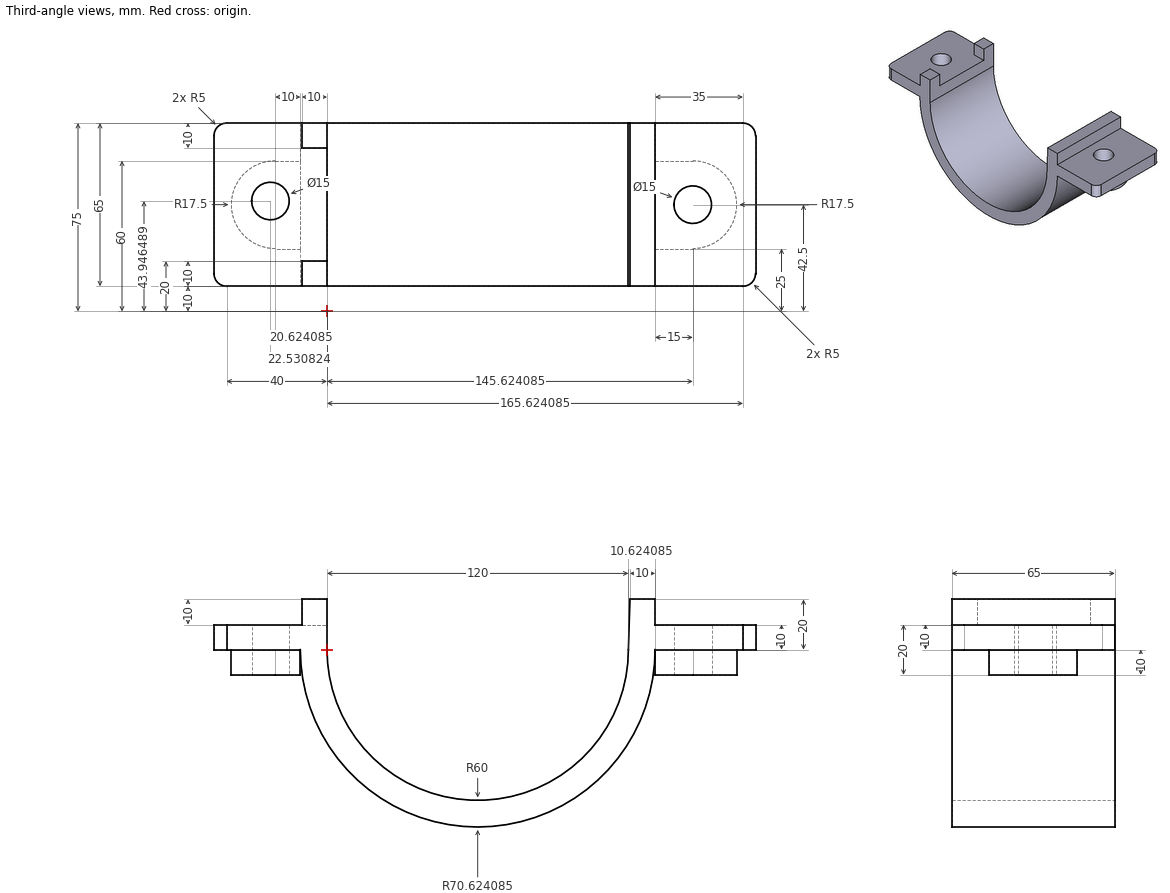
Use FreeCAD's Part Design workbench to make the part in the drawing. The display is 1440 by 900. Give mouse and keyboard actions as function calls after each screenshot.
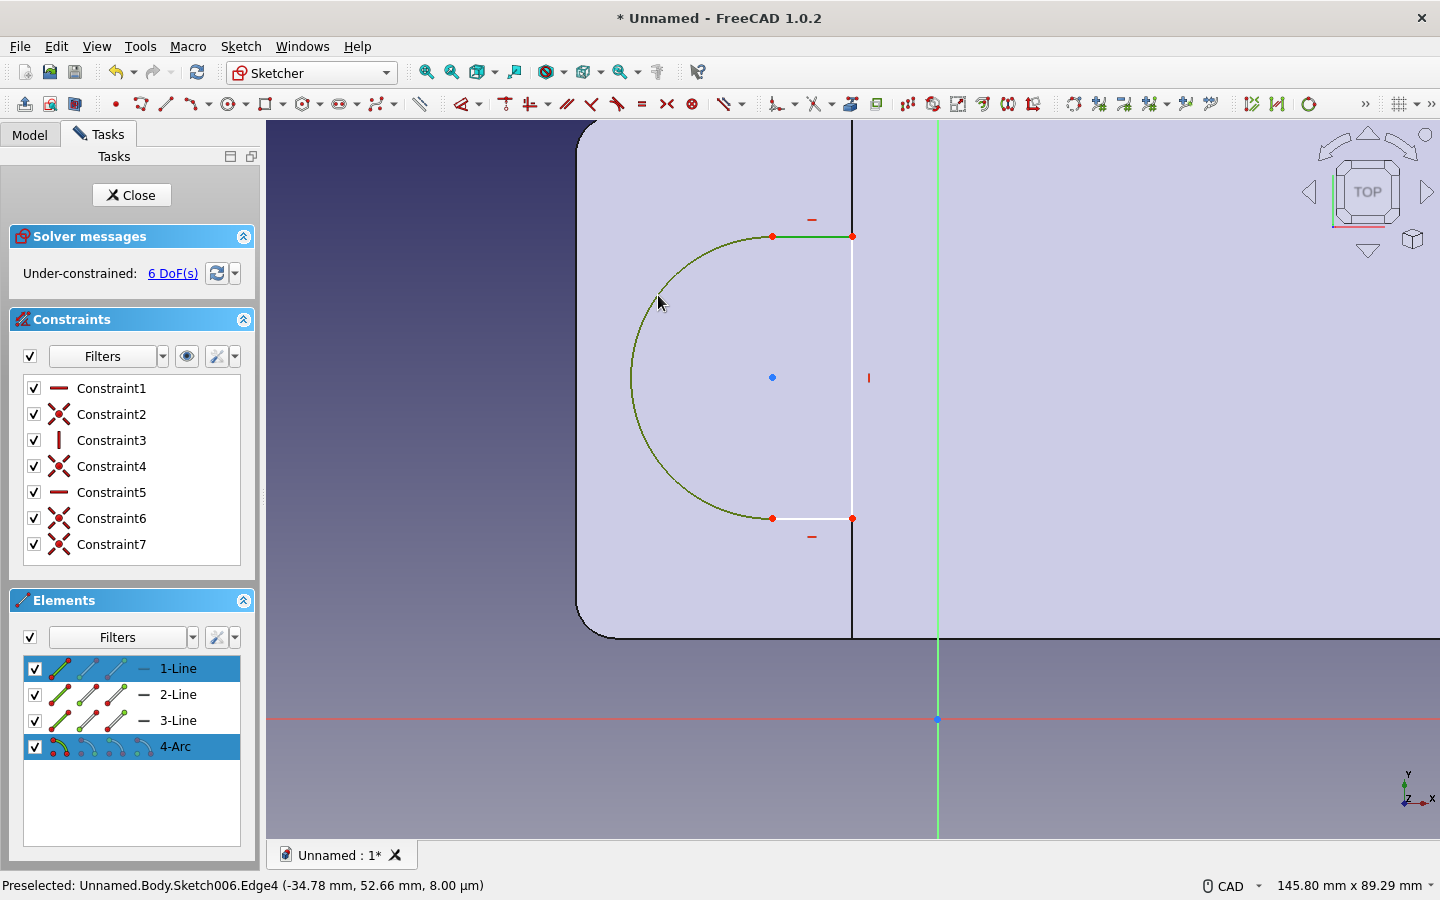
key(t)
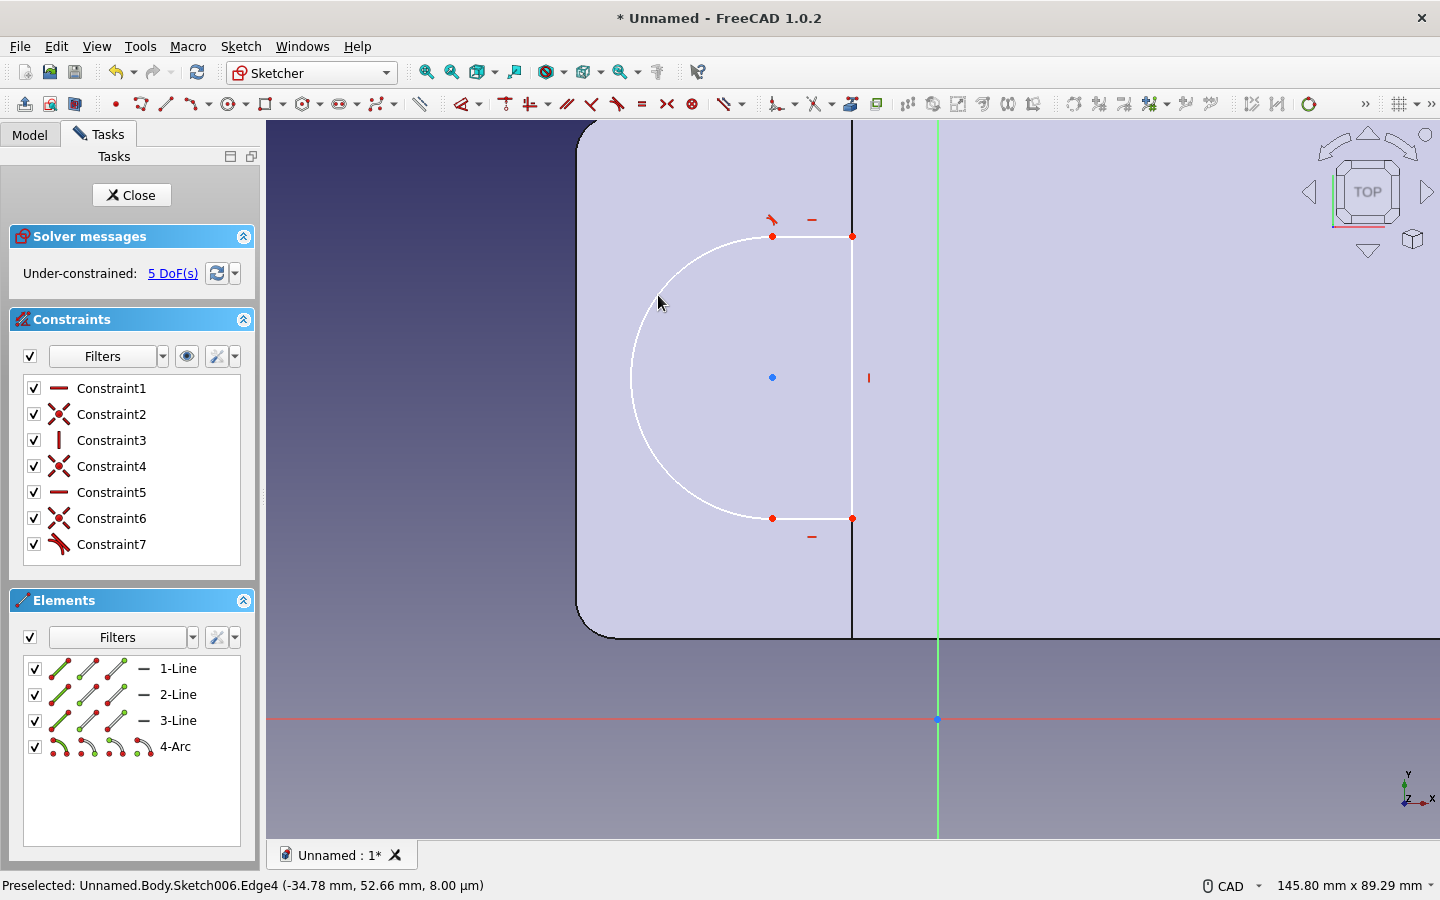
click(828, 519)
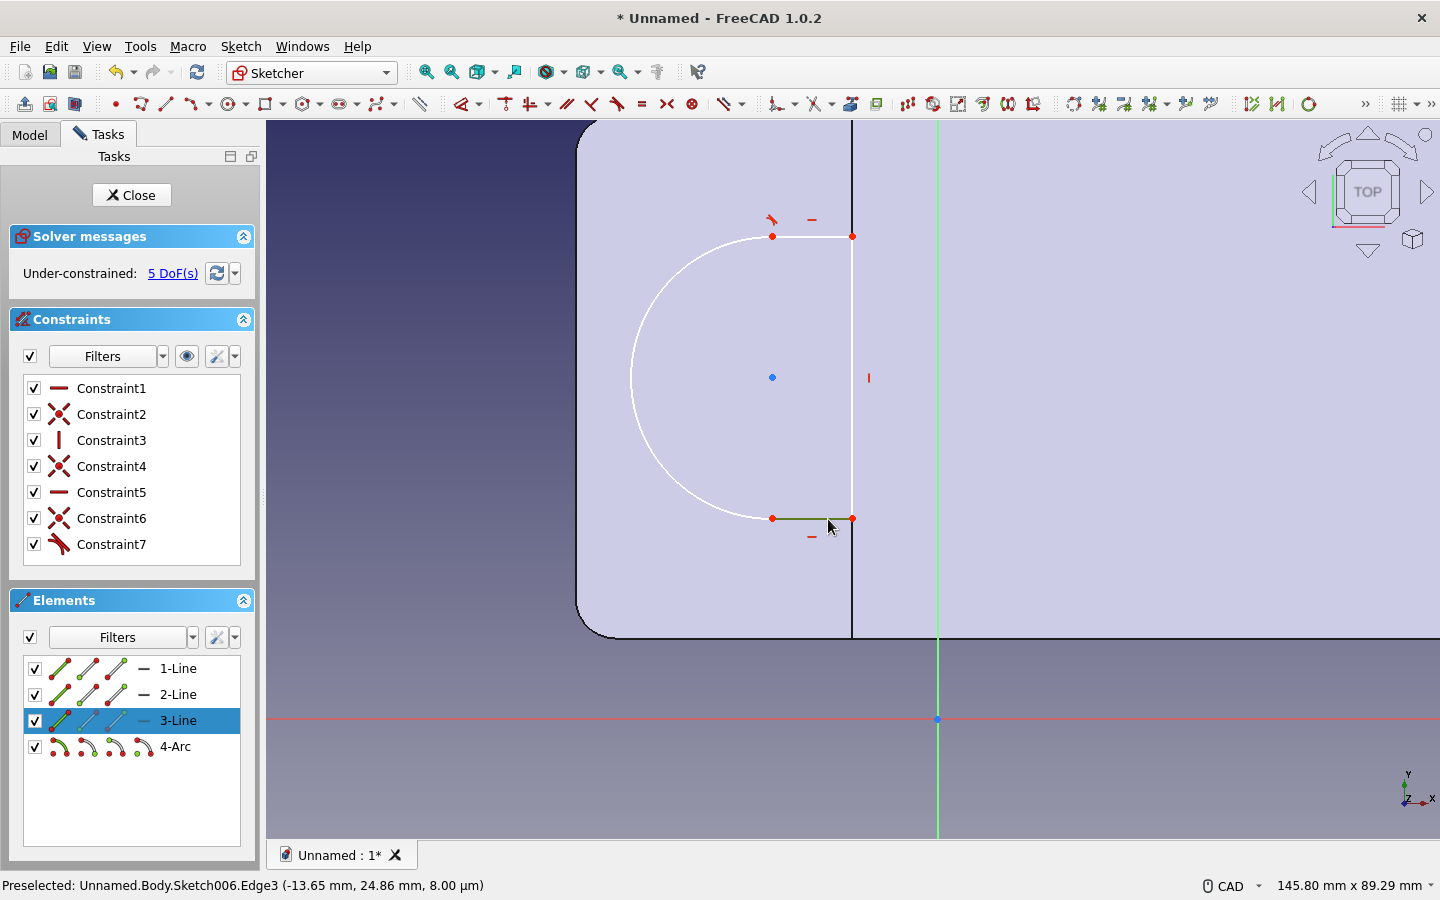
click(658, 295)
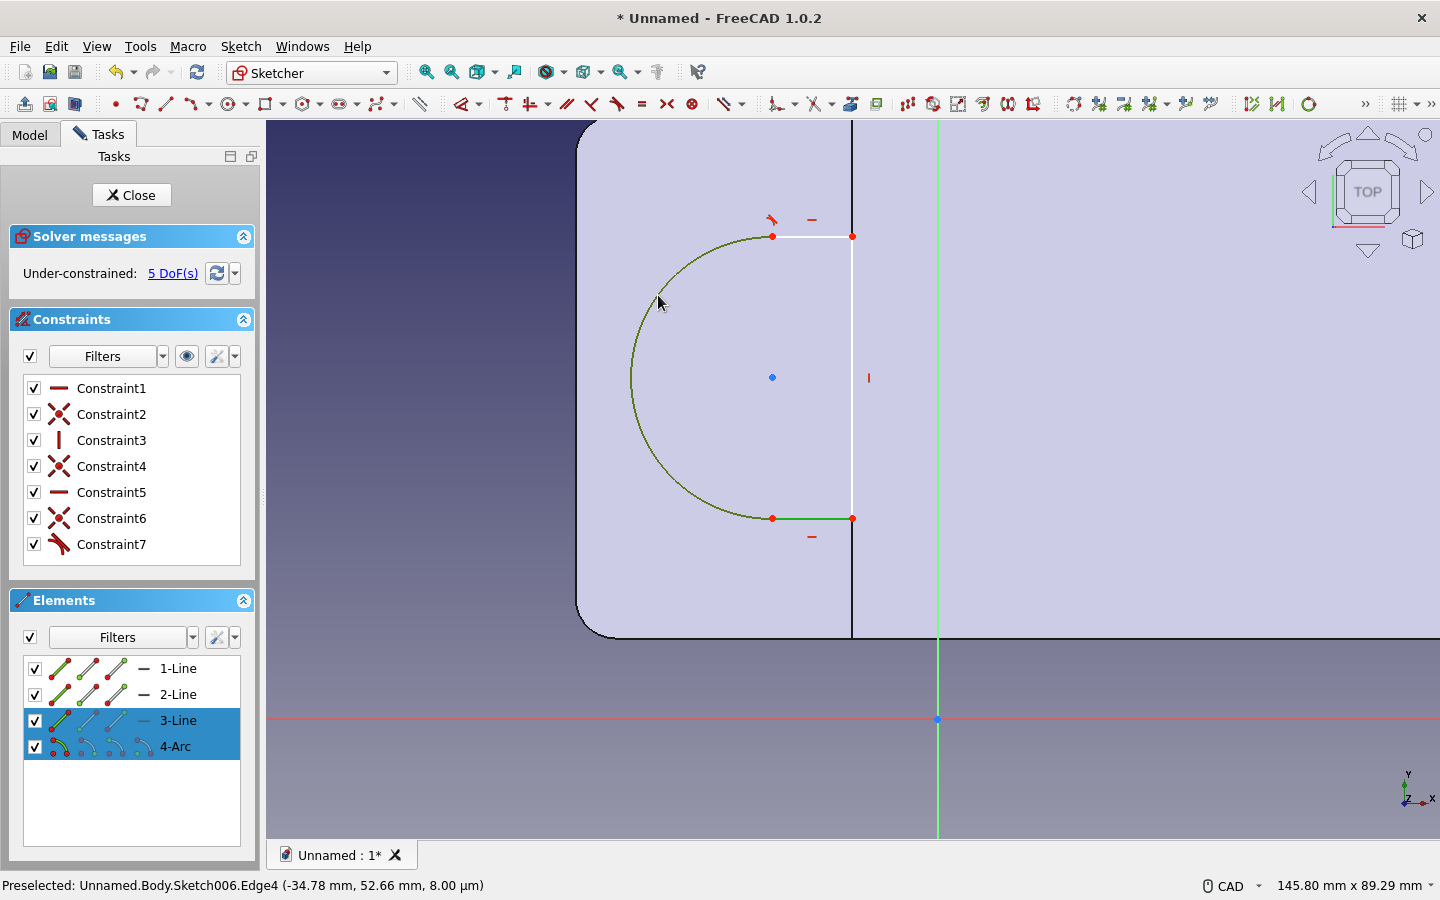
key(t)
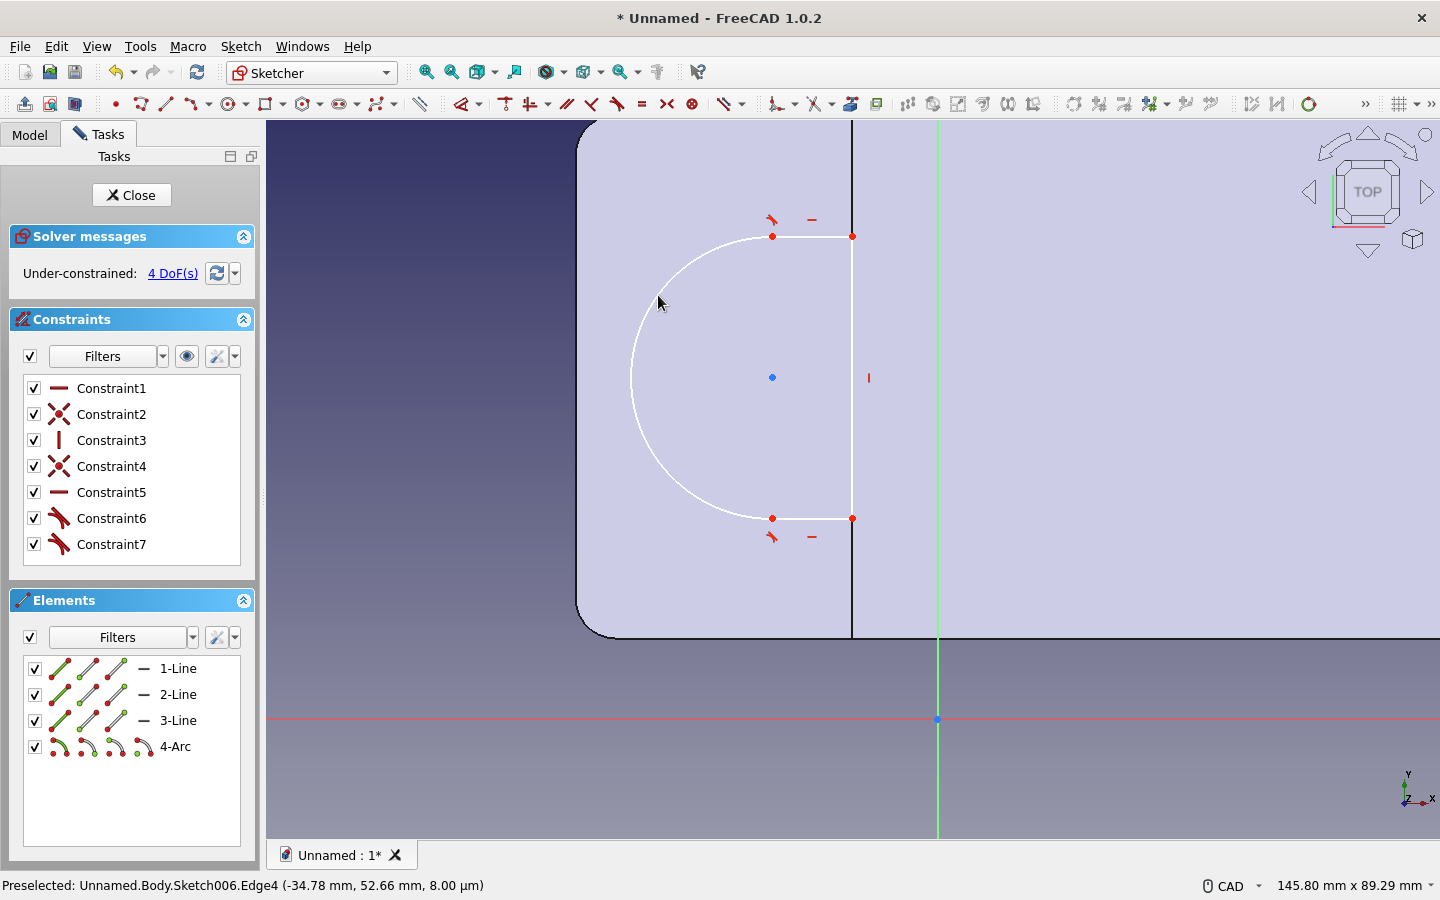
key(d)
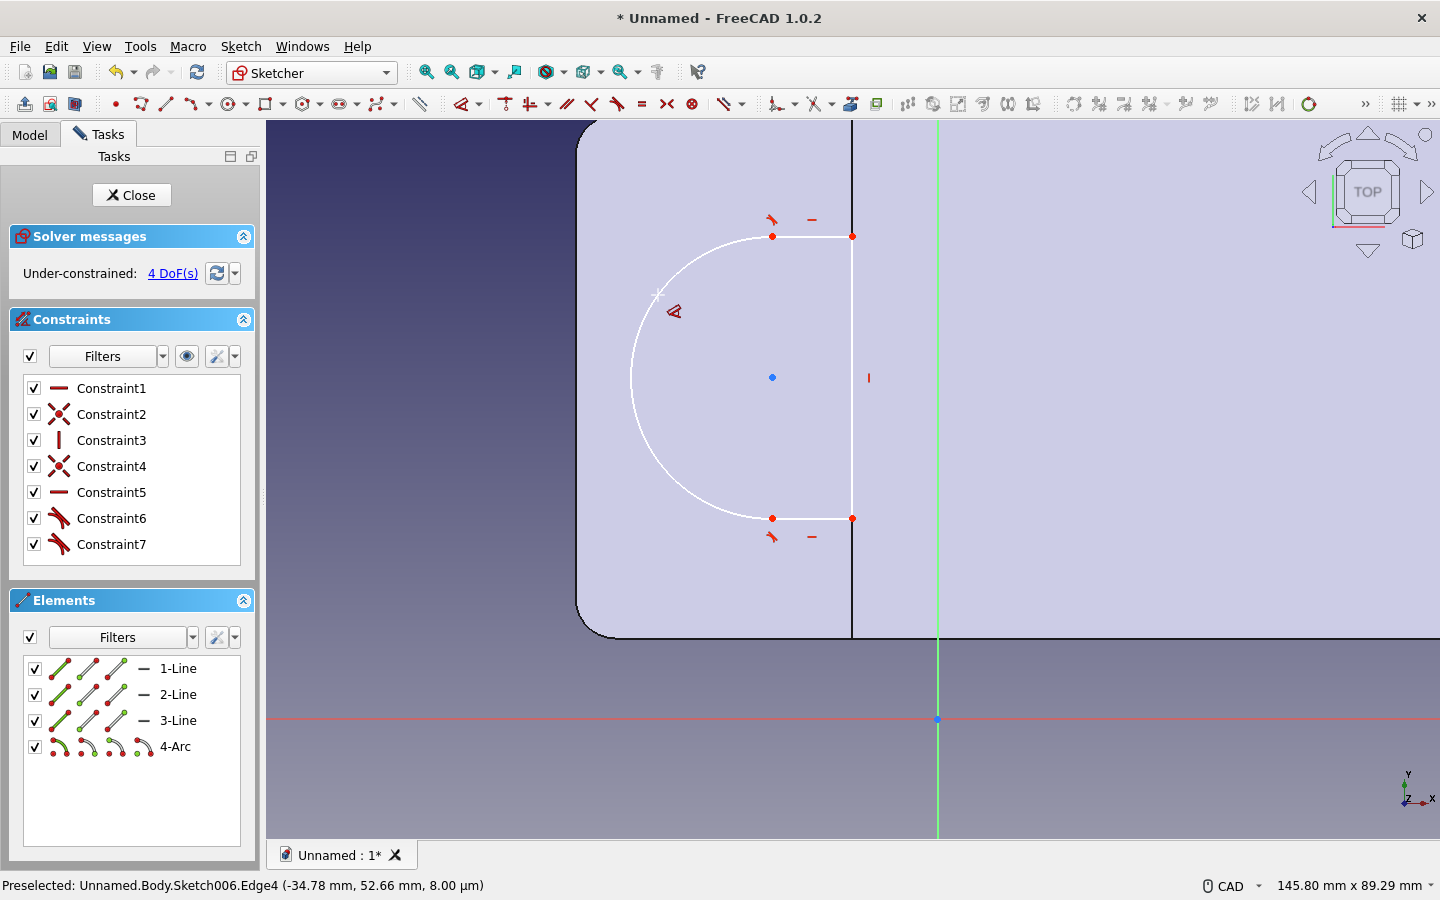
click(658, 295)
click(632, 276)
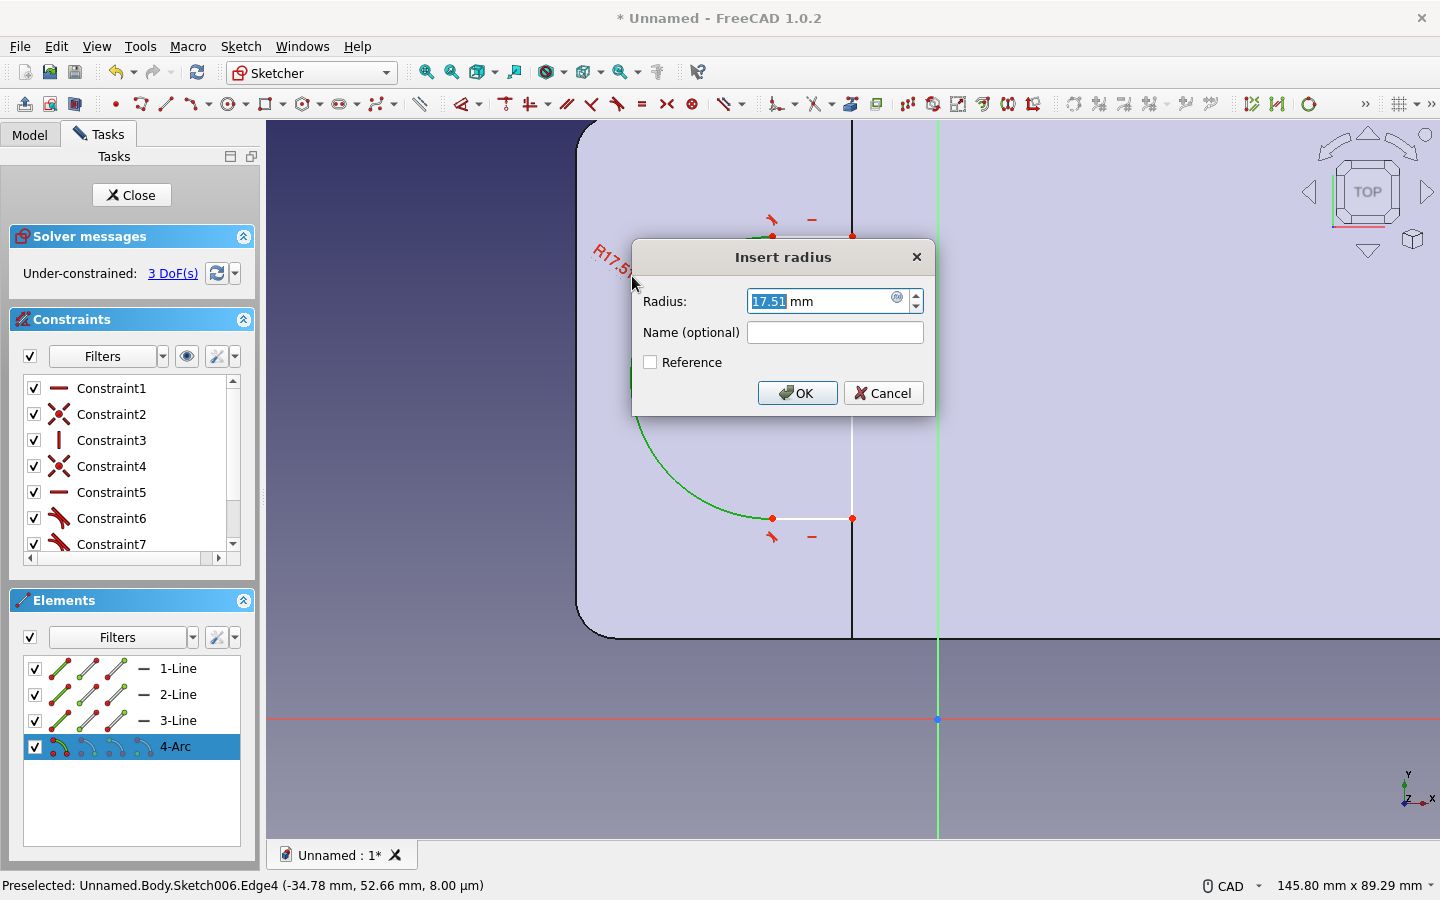
text(17.5)
key(Return)